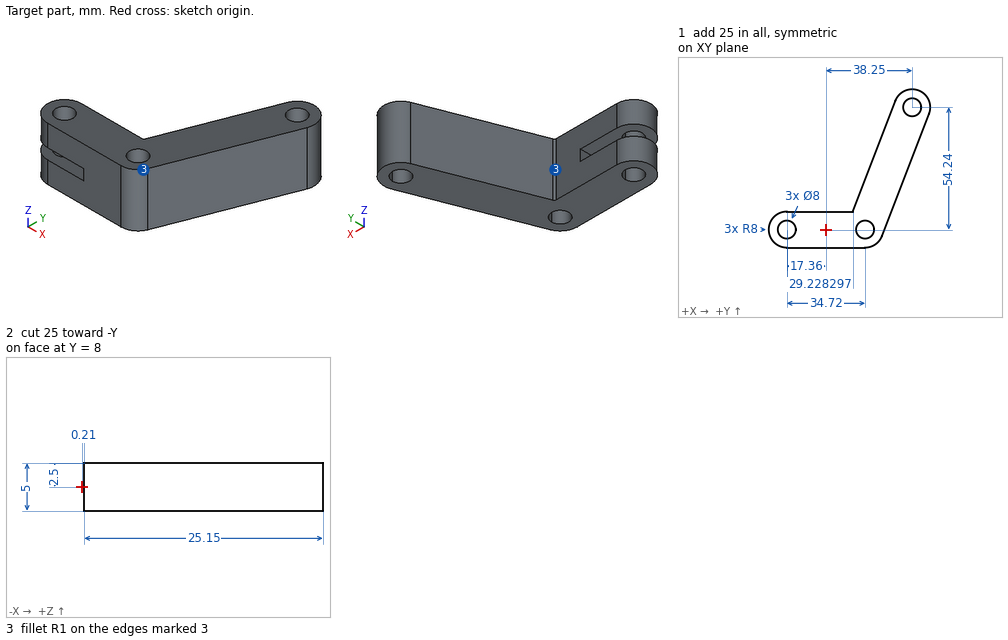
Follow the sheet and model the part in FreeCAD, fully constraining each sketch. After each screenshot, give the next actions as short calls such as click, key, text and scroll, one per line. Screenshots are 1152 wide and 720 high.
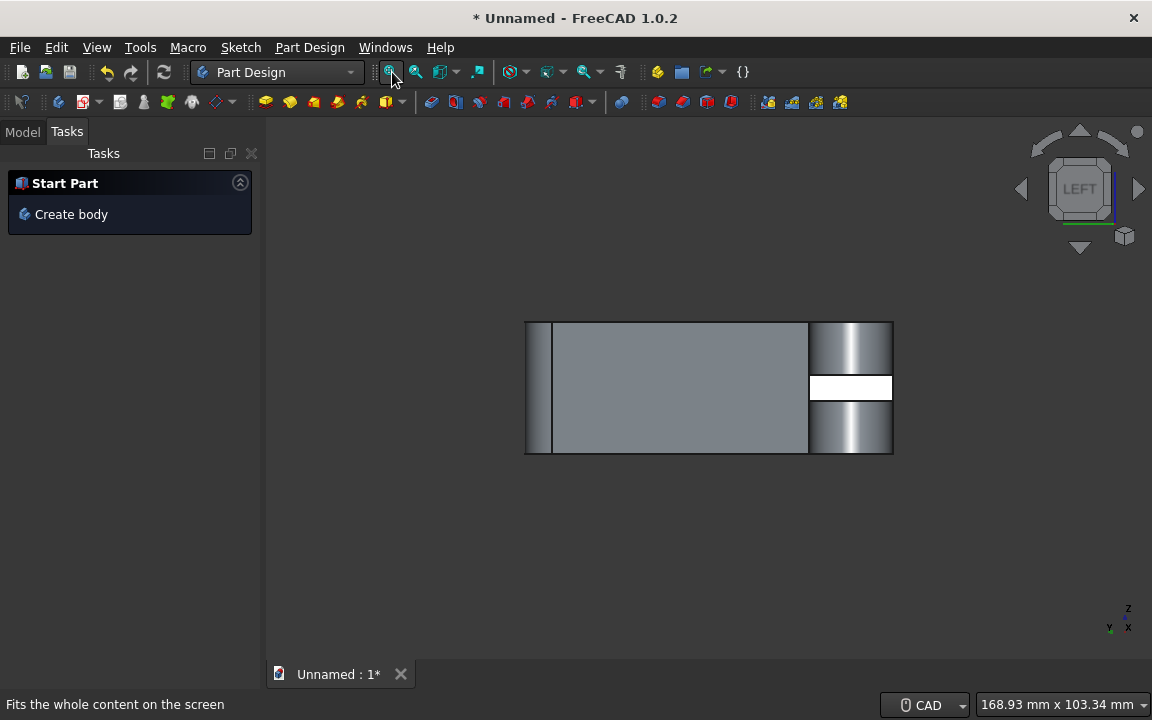
key(v)
key(3)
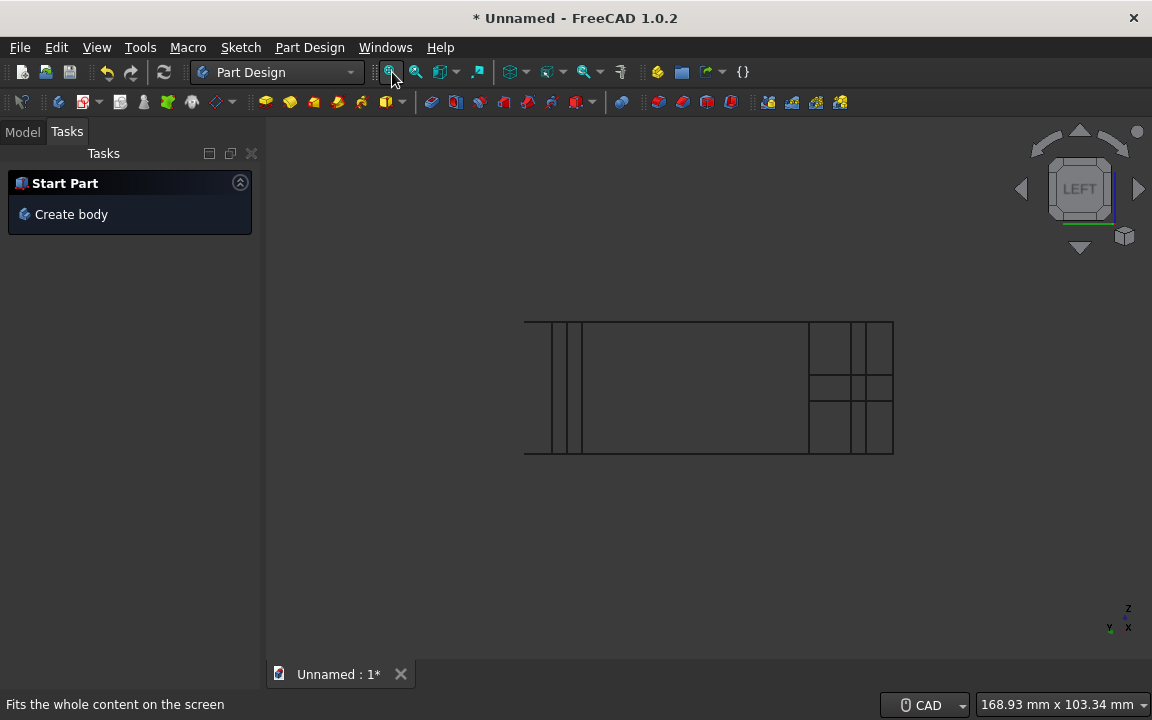
key(0)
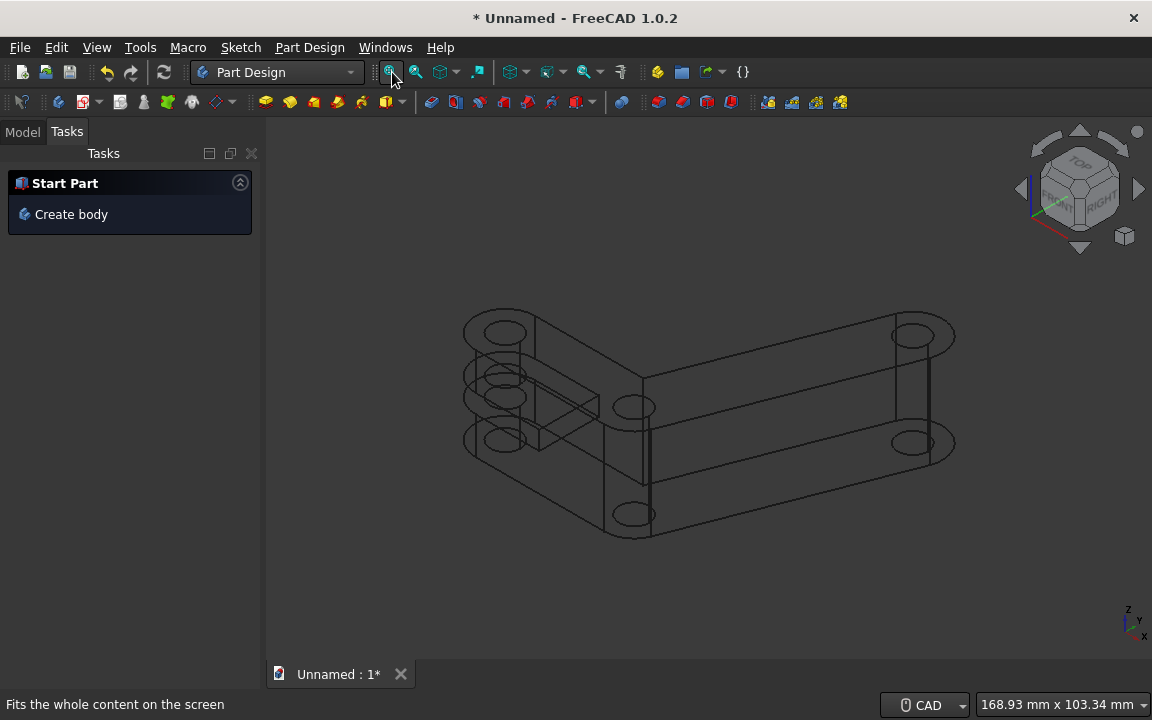
click(643, 410)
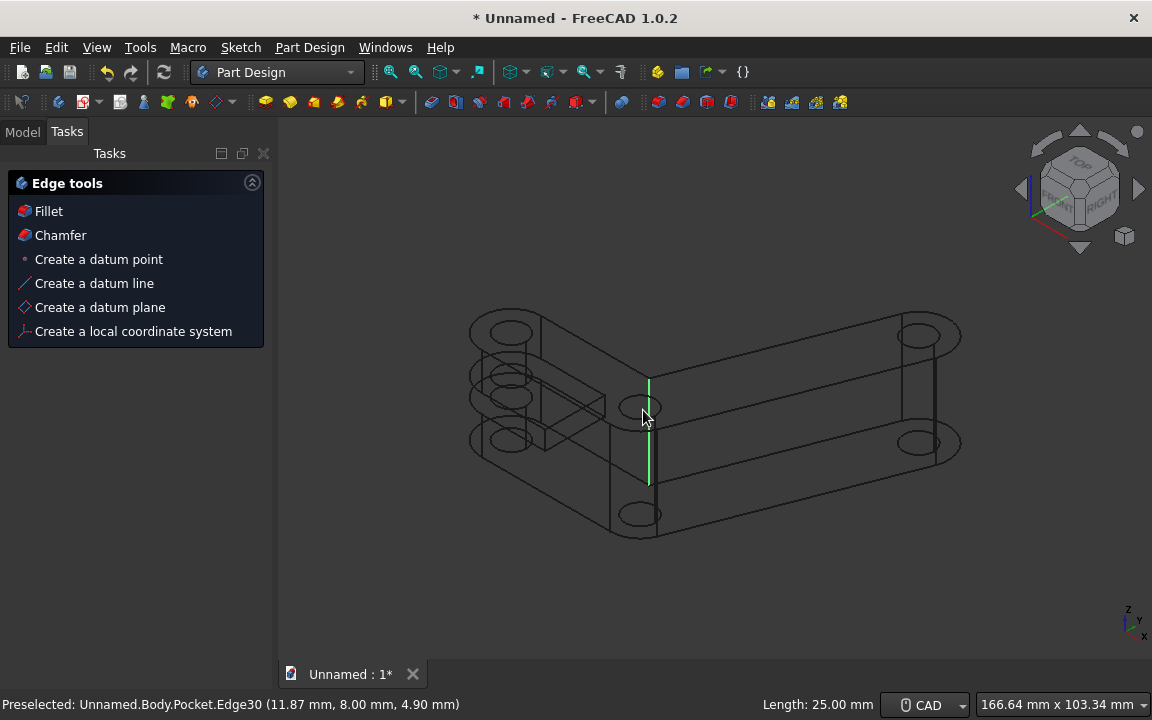
key(v)
key(1)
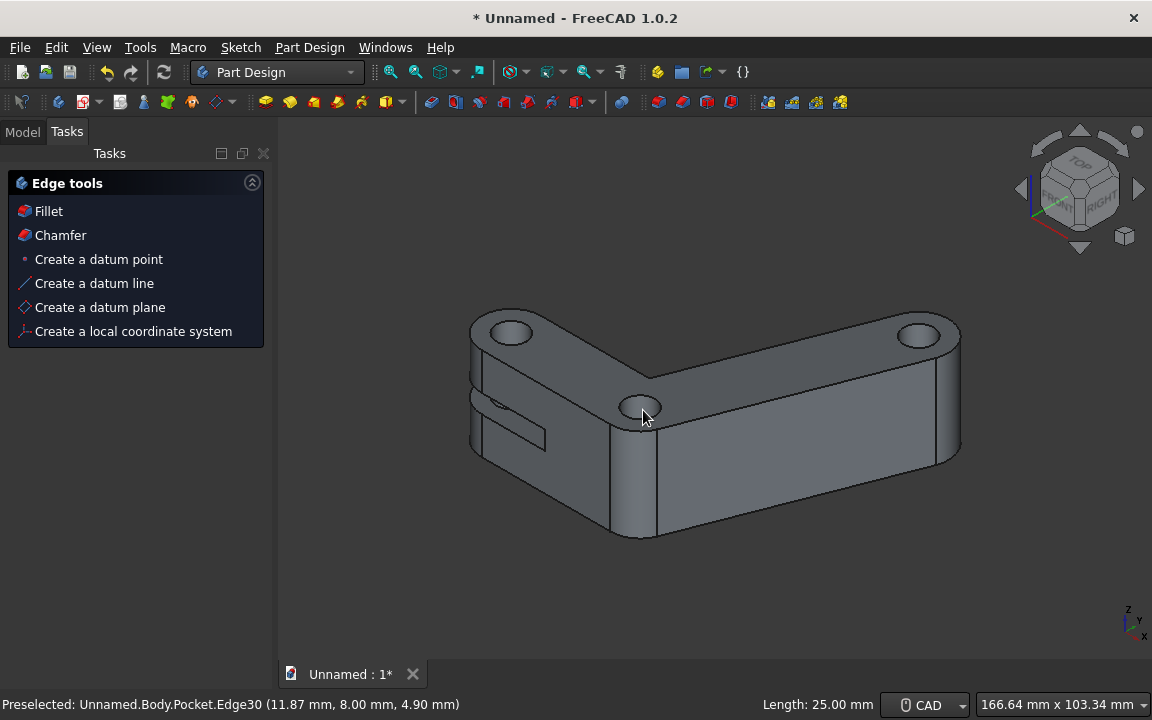
click(660, 102)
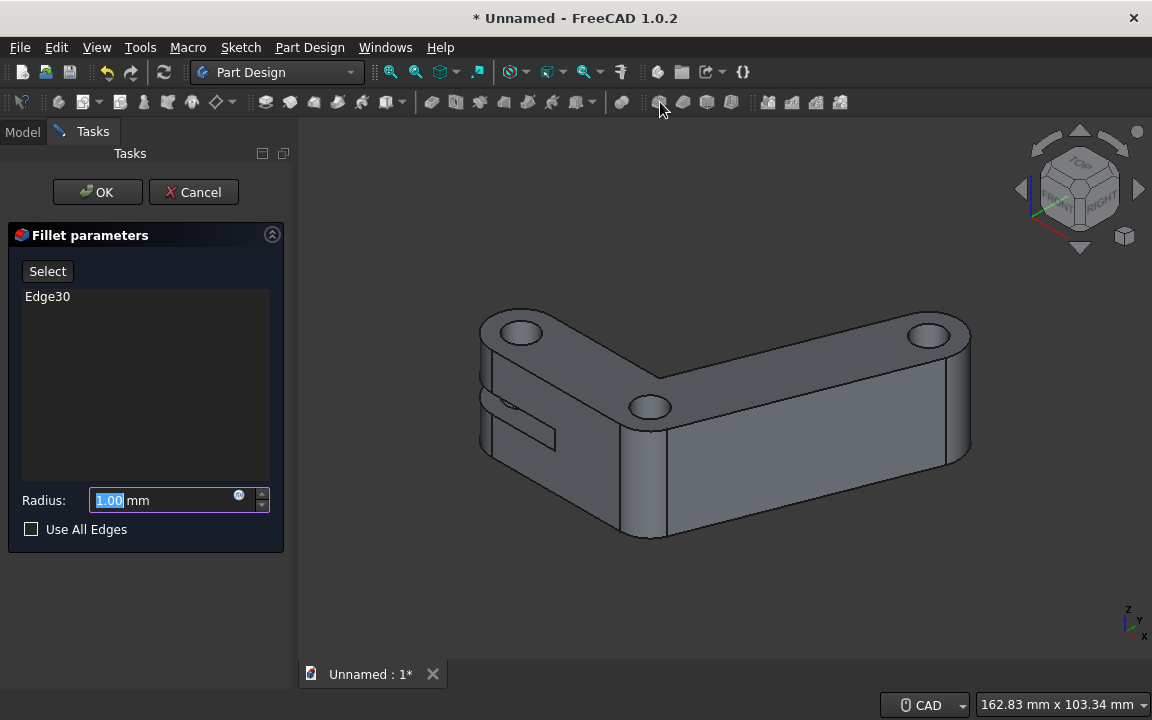
text(1)
key(Tab)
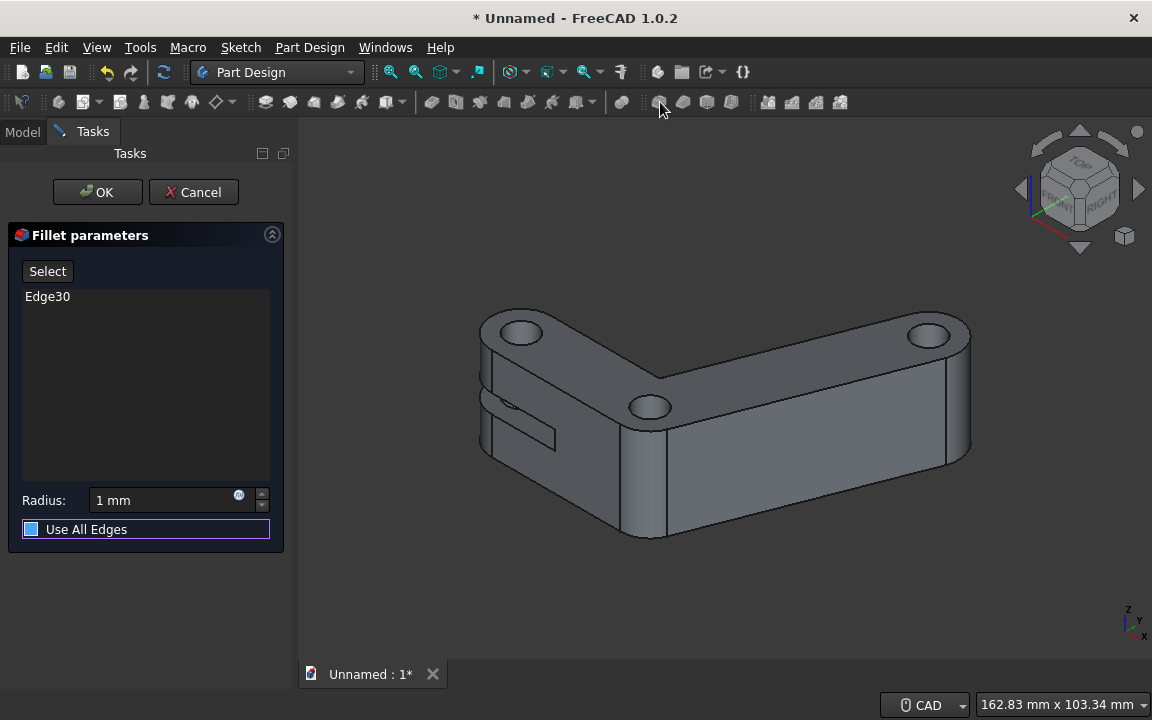
click(98, 192)